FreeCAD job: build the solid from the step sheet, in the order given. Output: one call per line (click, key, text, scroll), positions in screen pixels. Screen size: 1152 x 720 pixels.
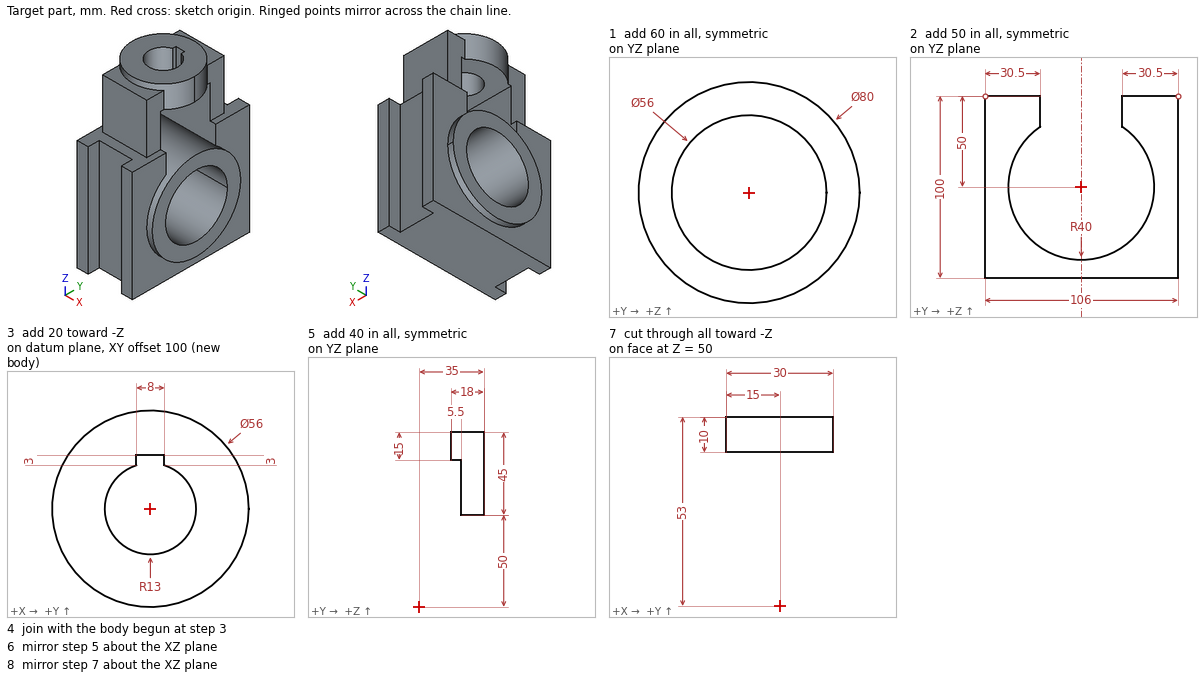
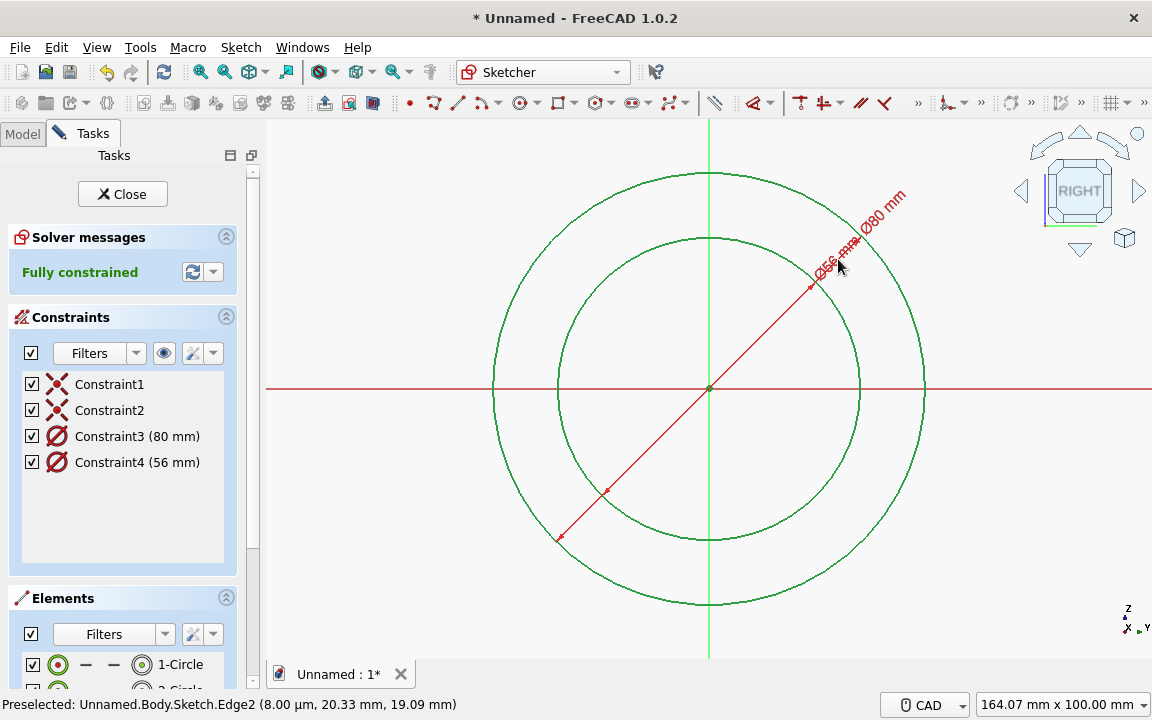
click(123, 194)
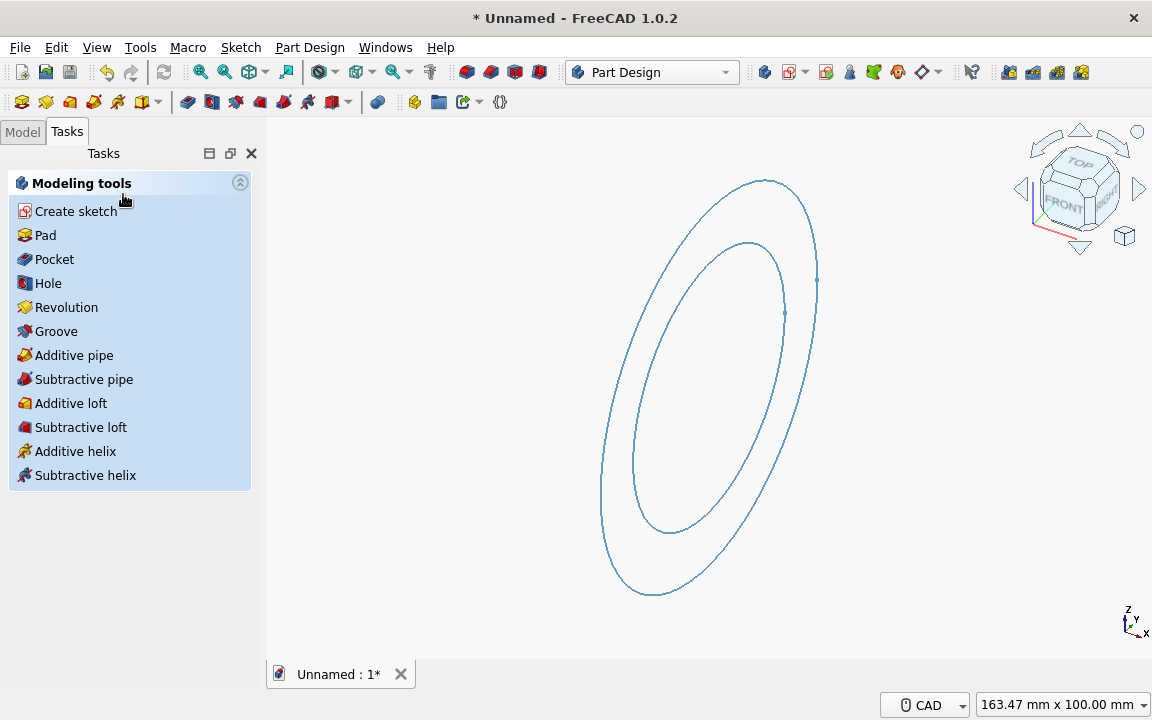
click(22, 102)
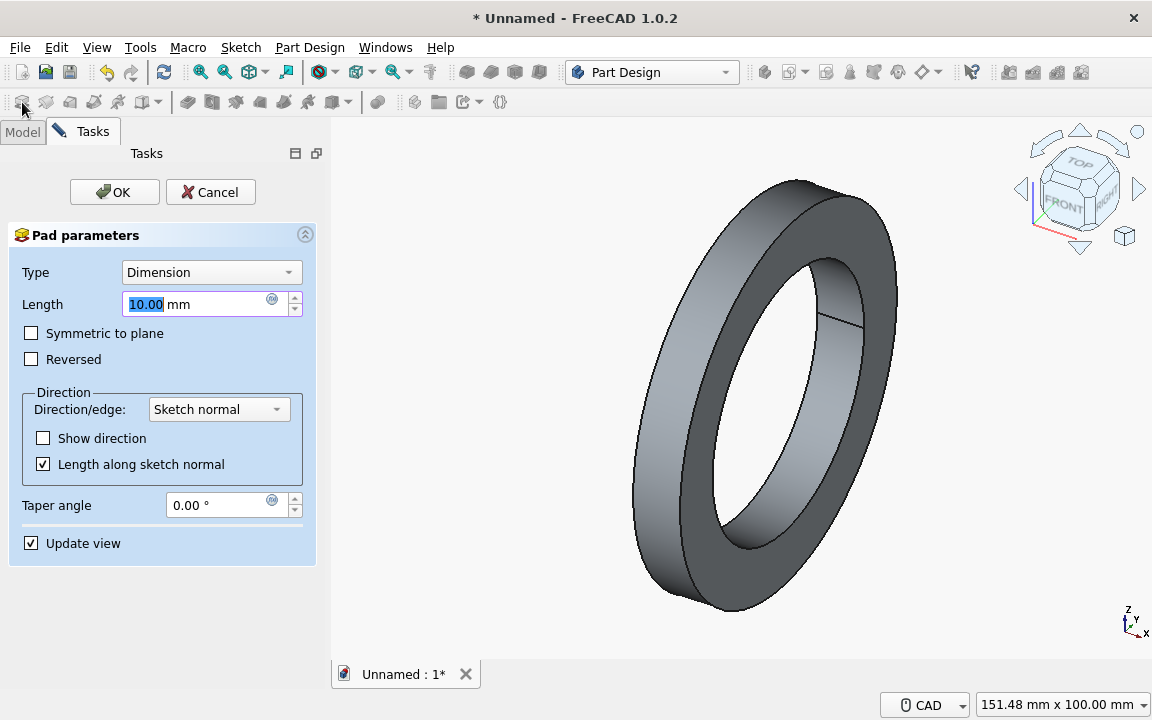
text(60)
key(Tab)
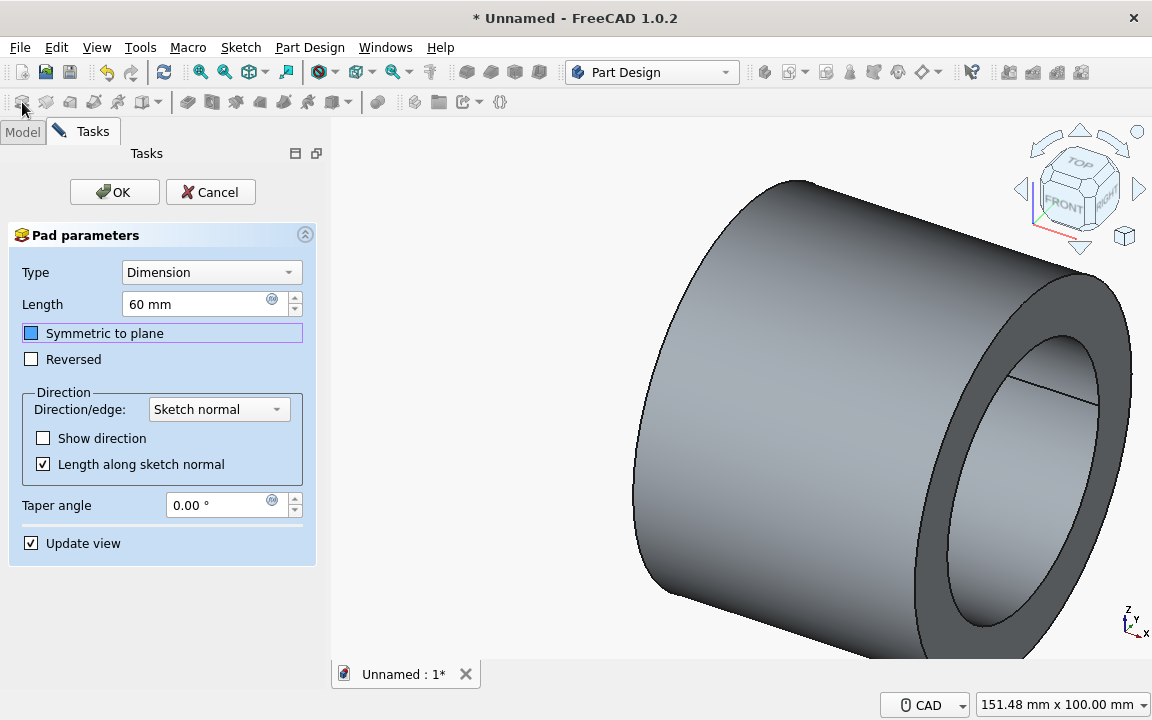
click(30, 333)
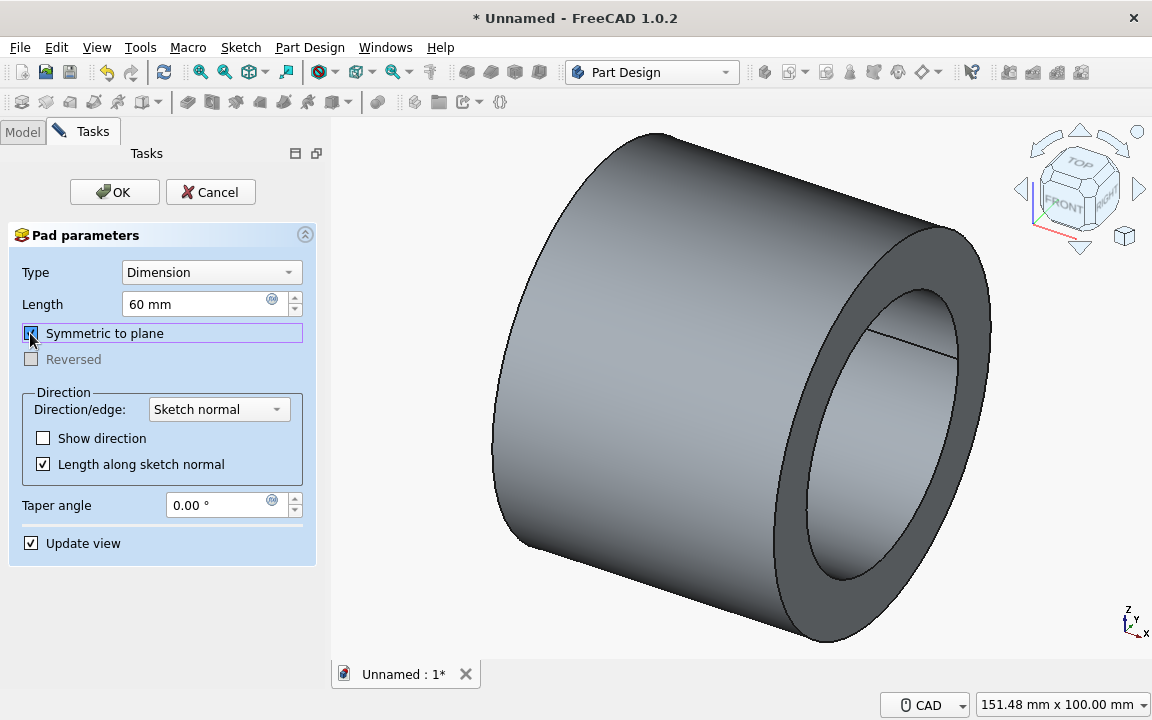
click(115, 192)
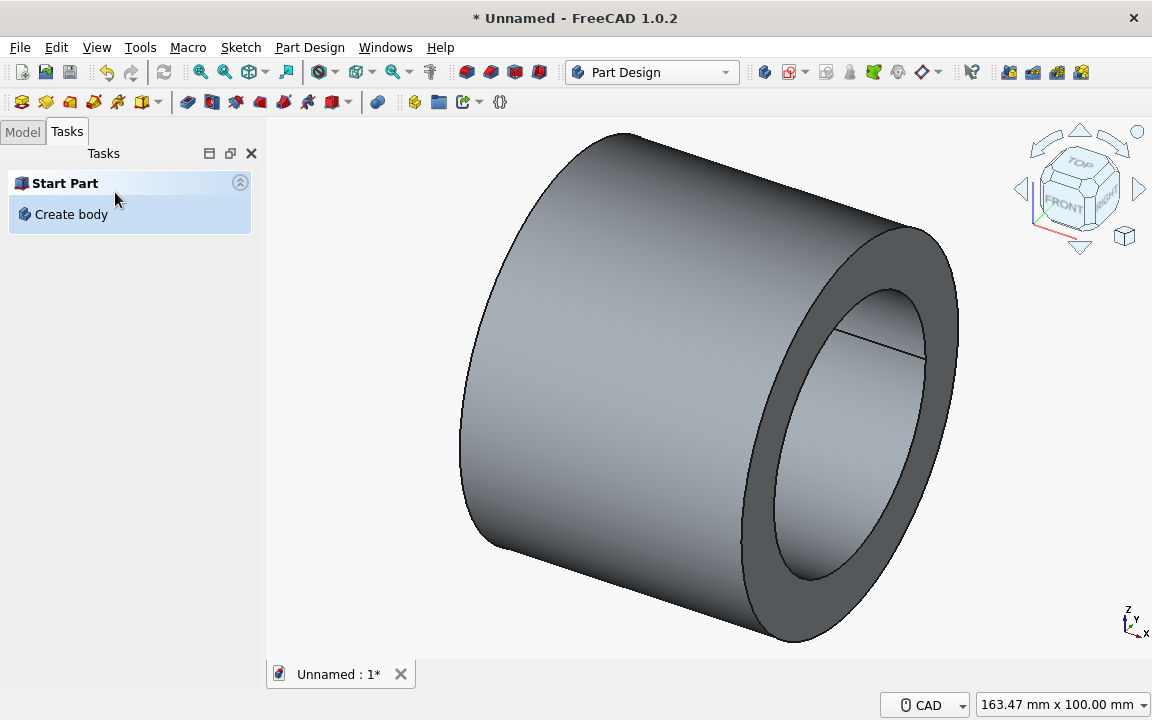
click(202, 72)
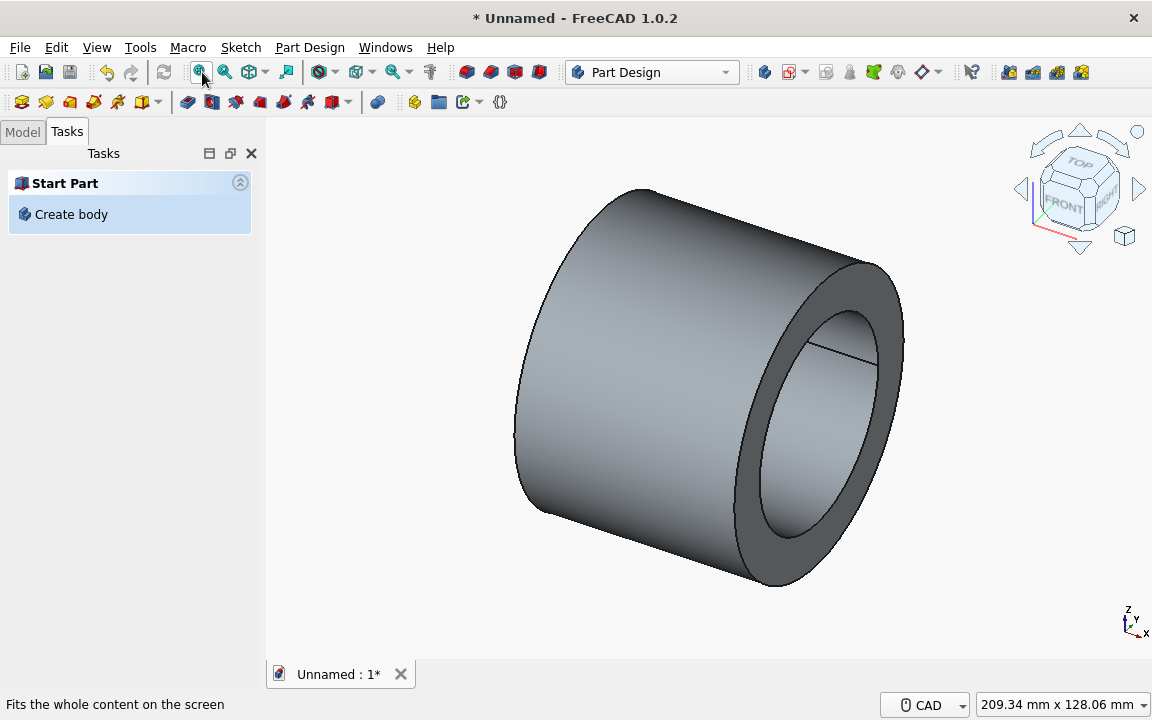
click(790, 72)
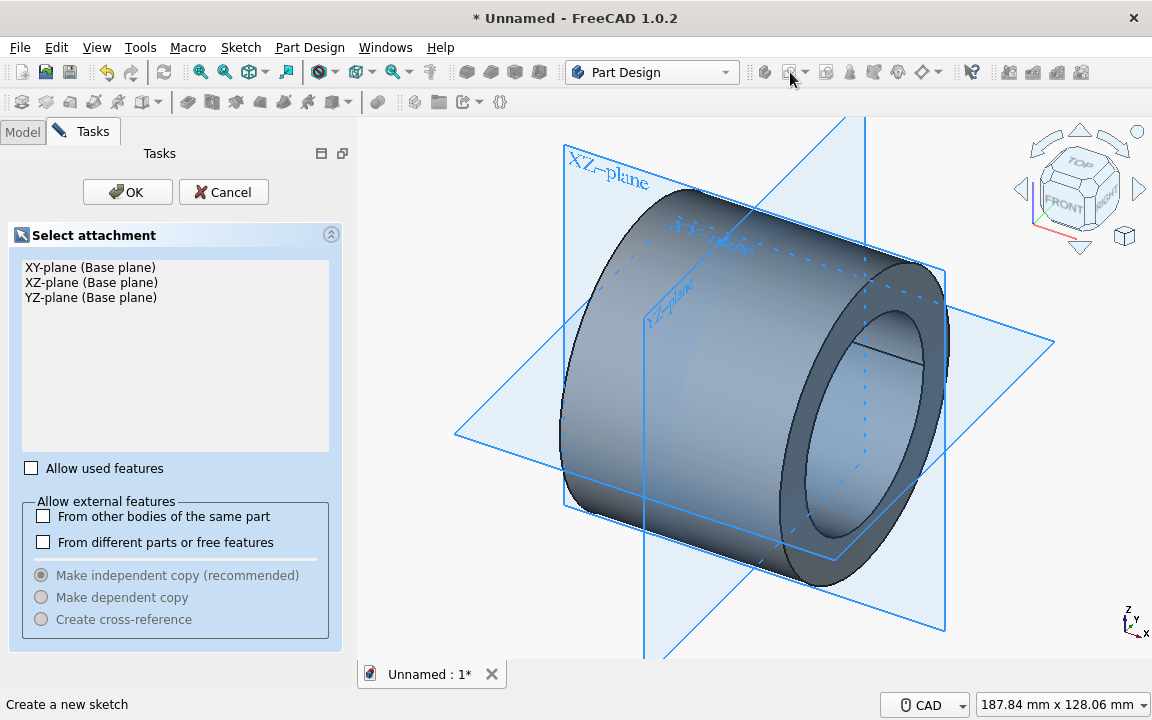
click(82, 298)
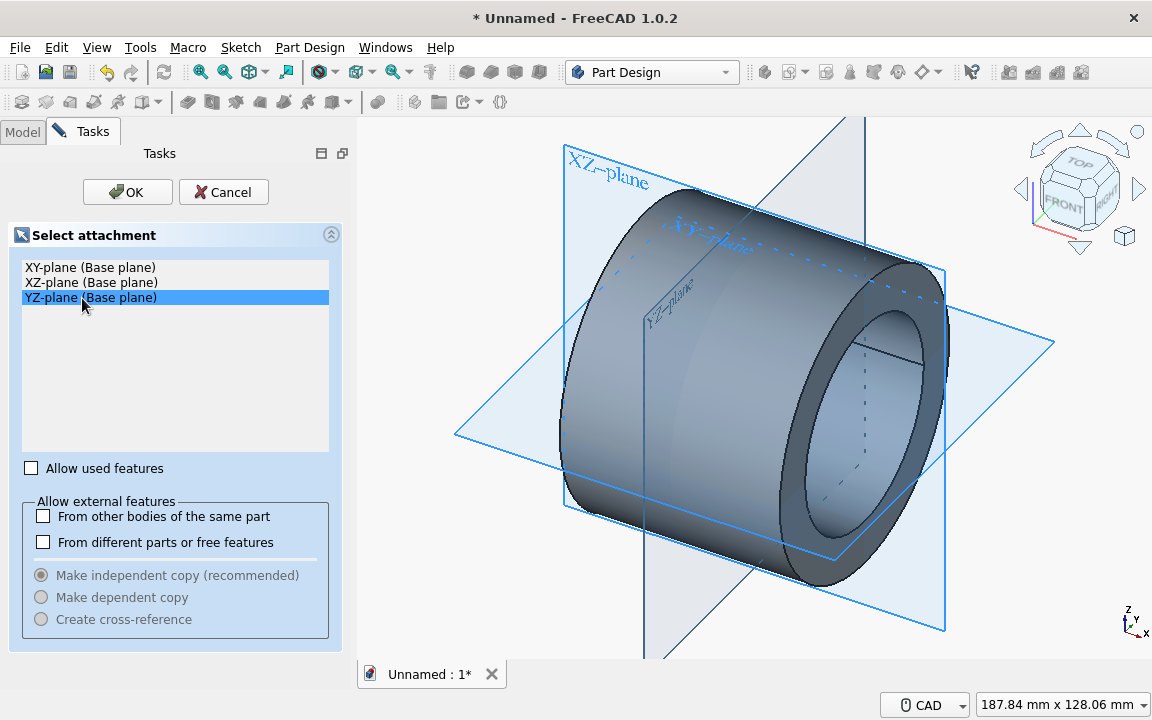
click(128, 192)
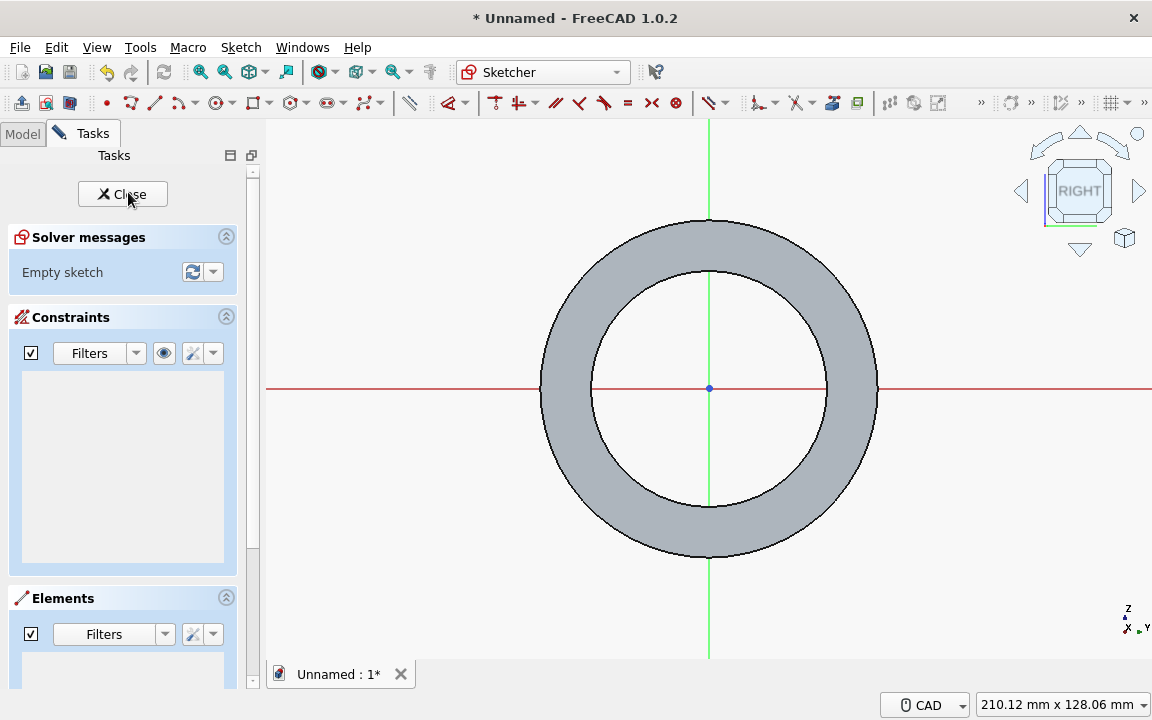
click(70, 104)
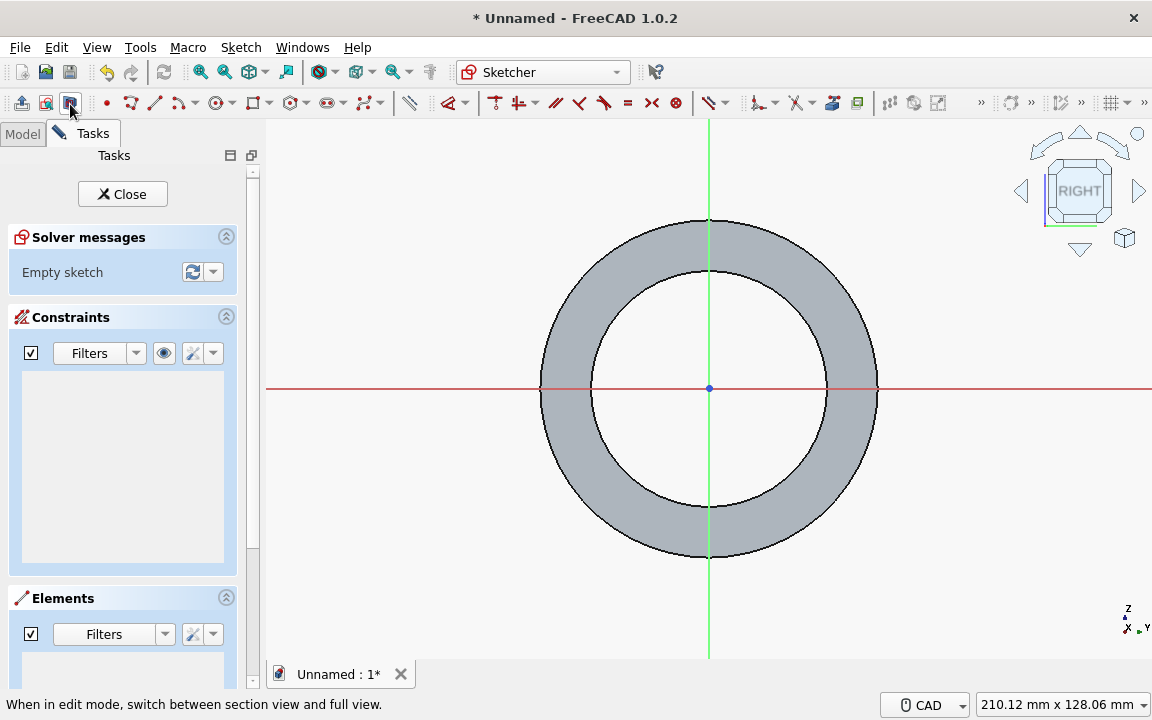
click(132, 104)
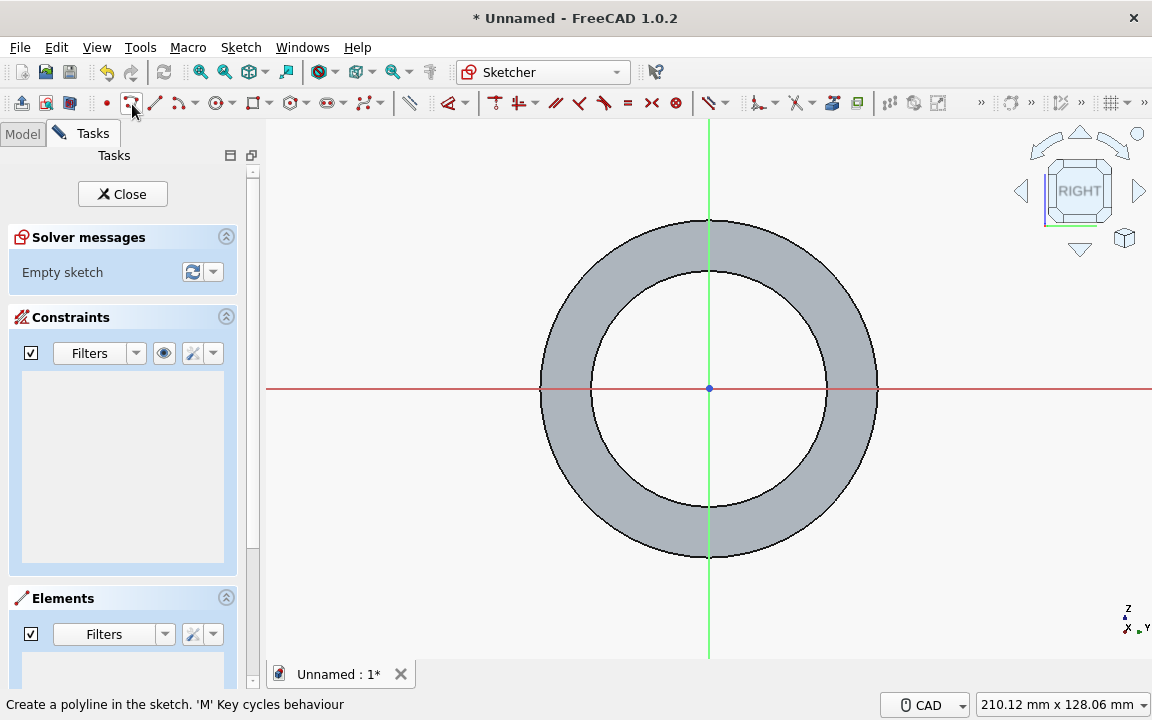
click(614, 250)
click(614, 178)
click(486, 178)
click(486, 600)
click(932, 600)
click(932, 178)
click(804, 178)
click(804, 250)
right_click(804, 250)